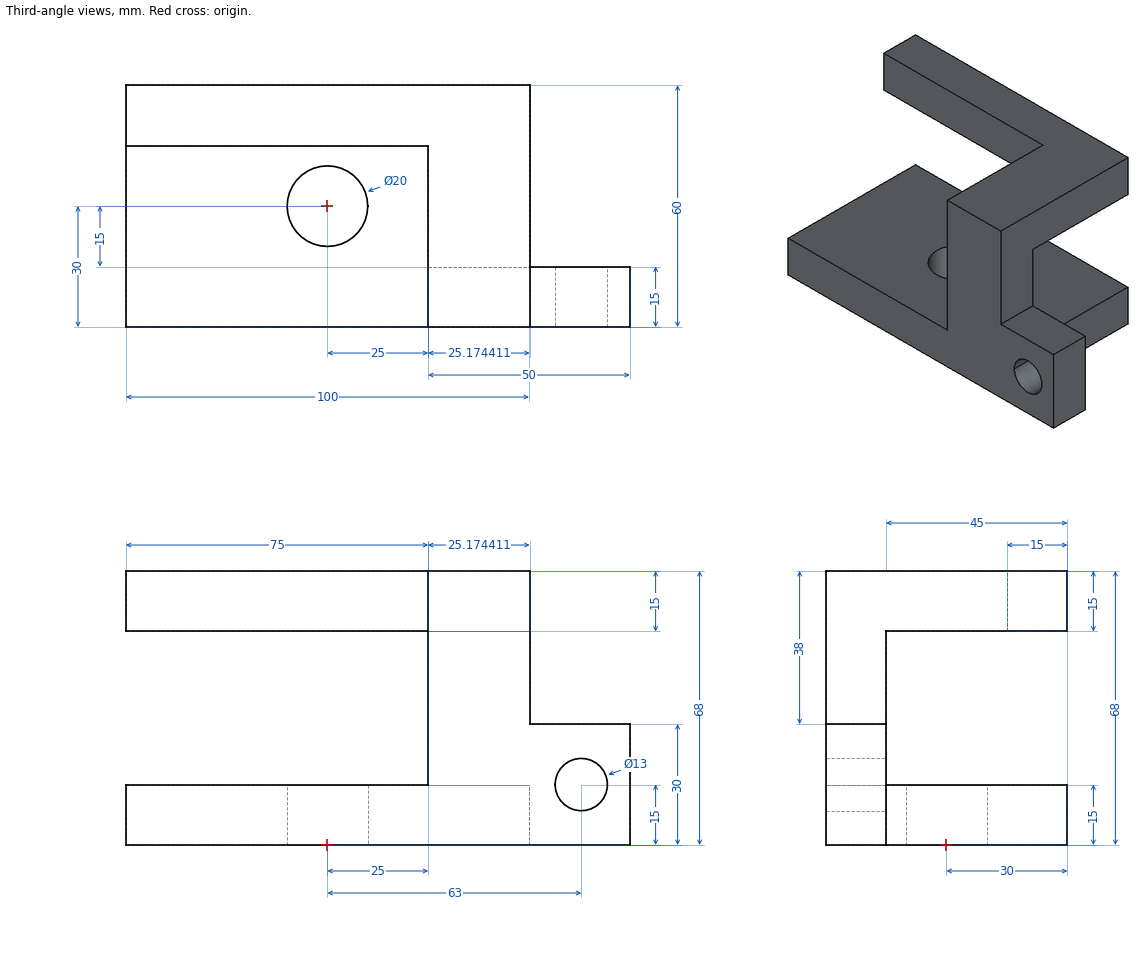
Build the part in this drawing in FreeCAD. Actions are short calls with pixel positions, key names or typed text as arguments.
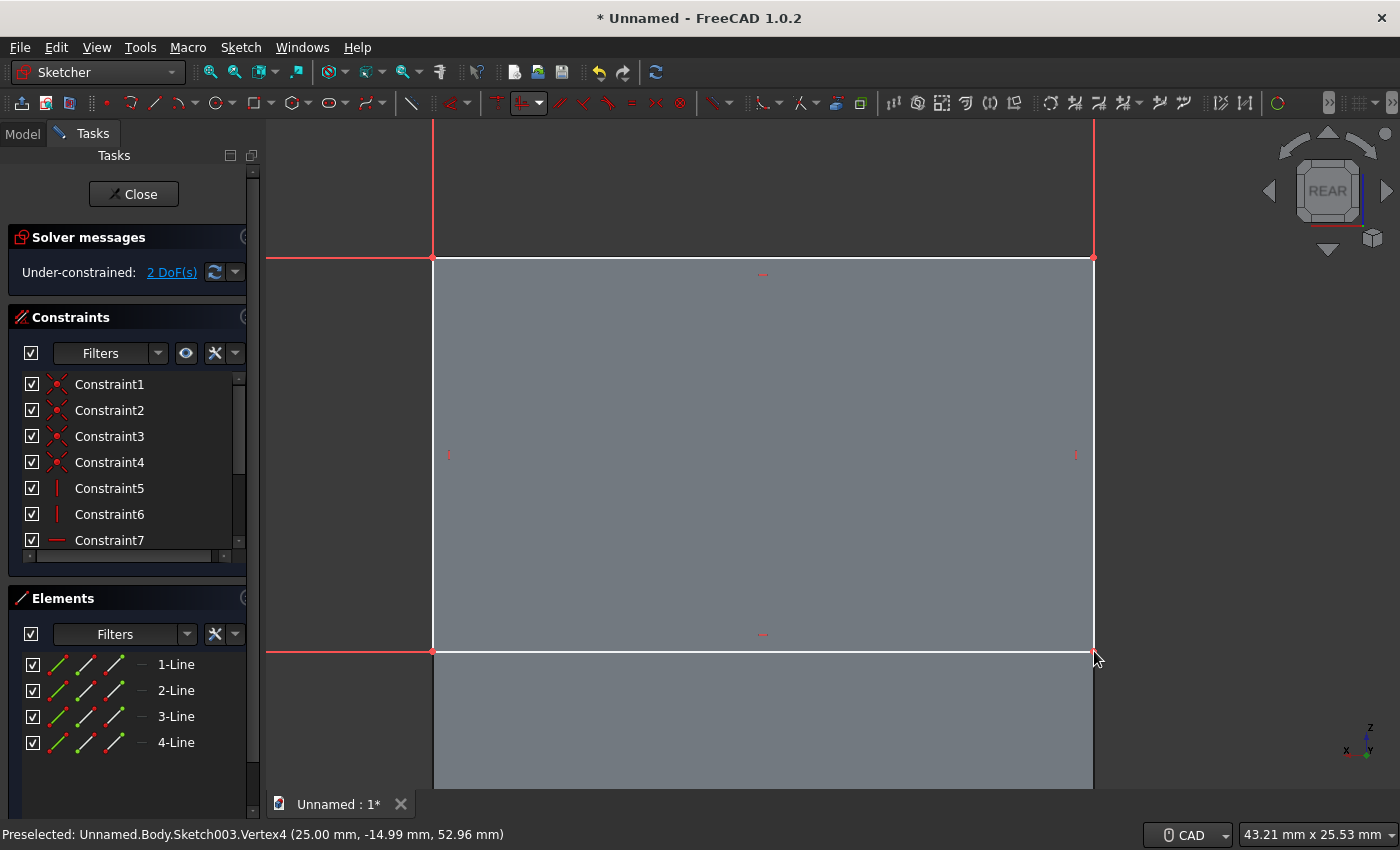
click(450, 104)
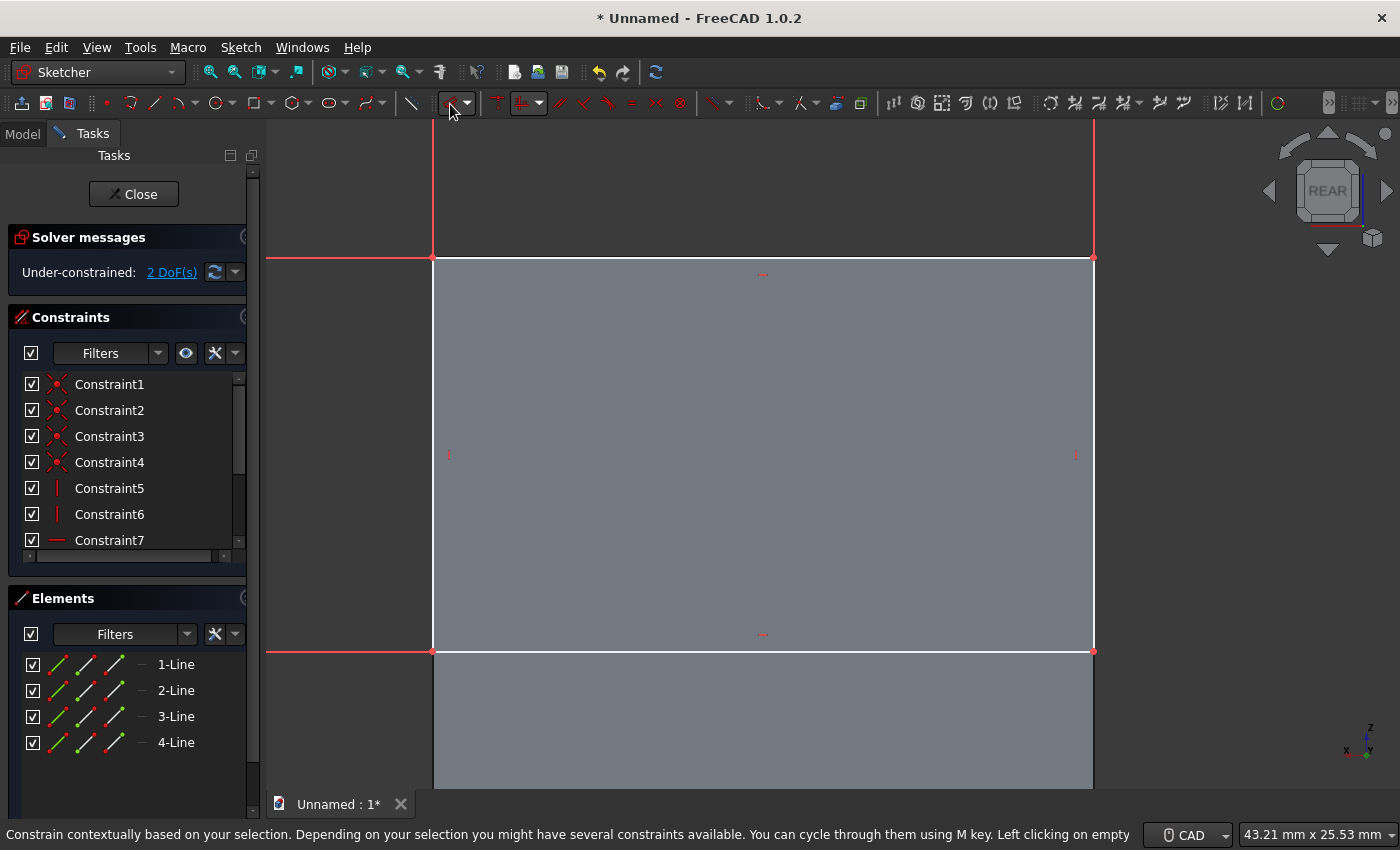
click(433, 258)
click(399, 510)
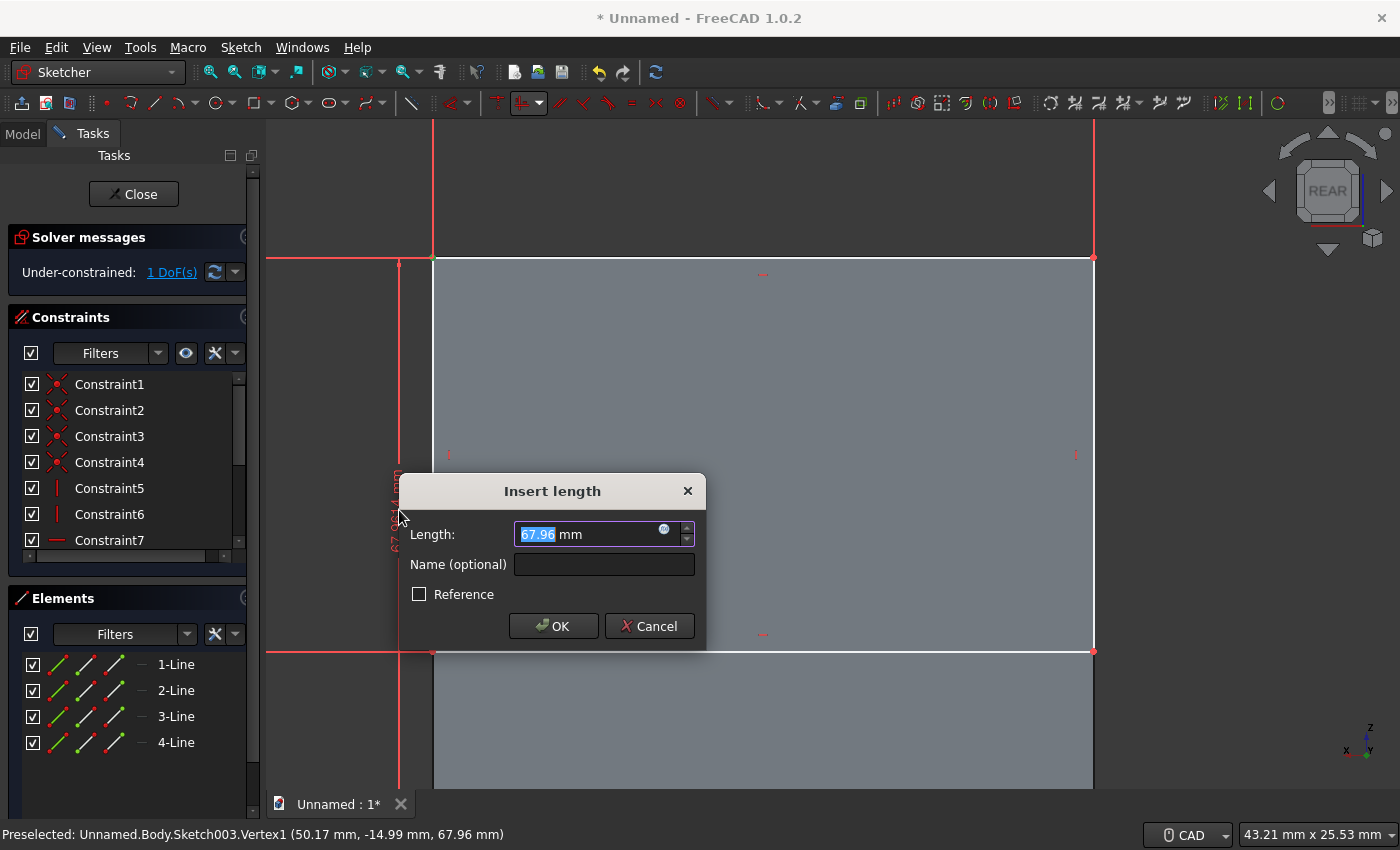
text(68)
key(Return)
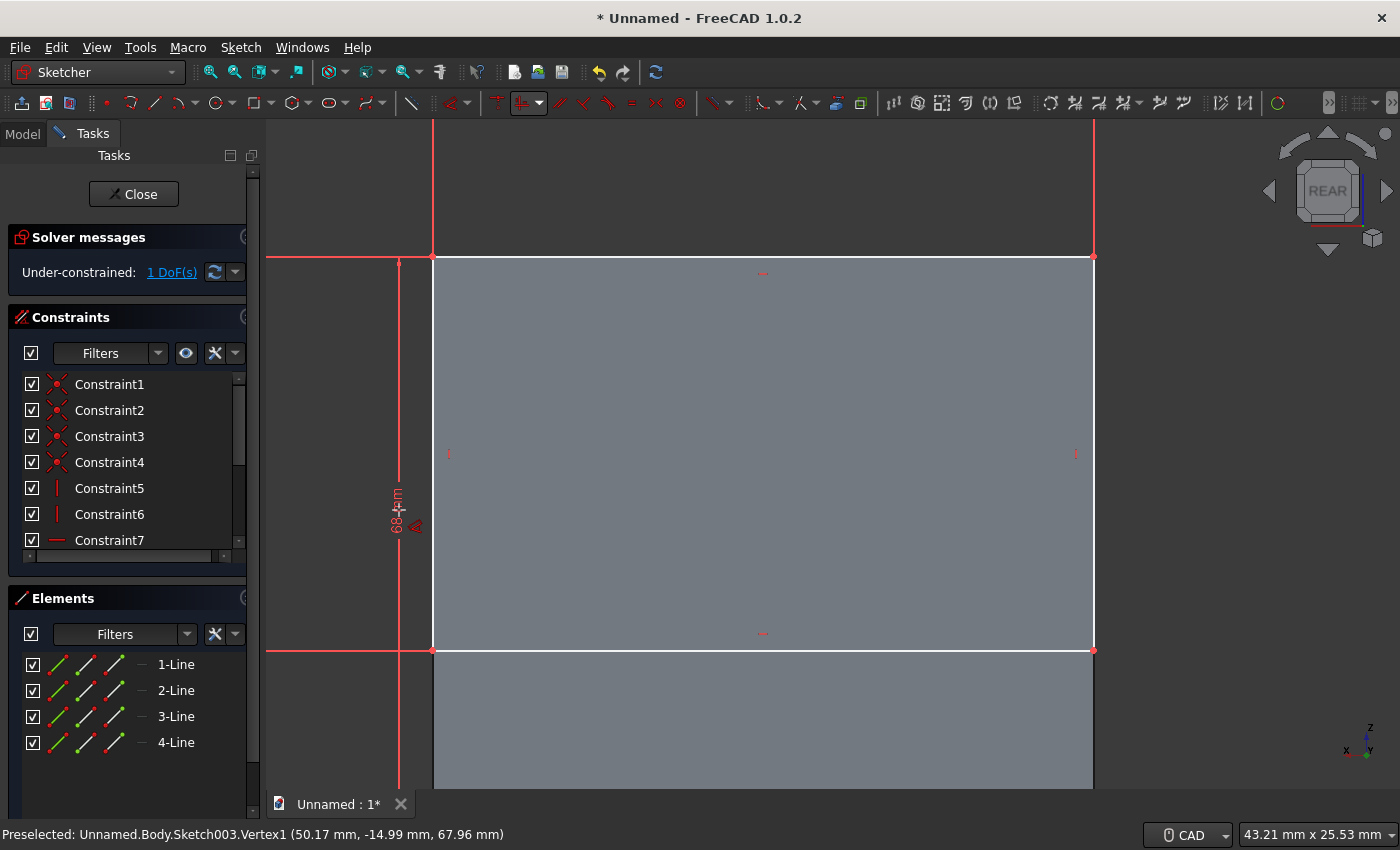
click(1094, 651)
click(1164, 617)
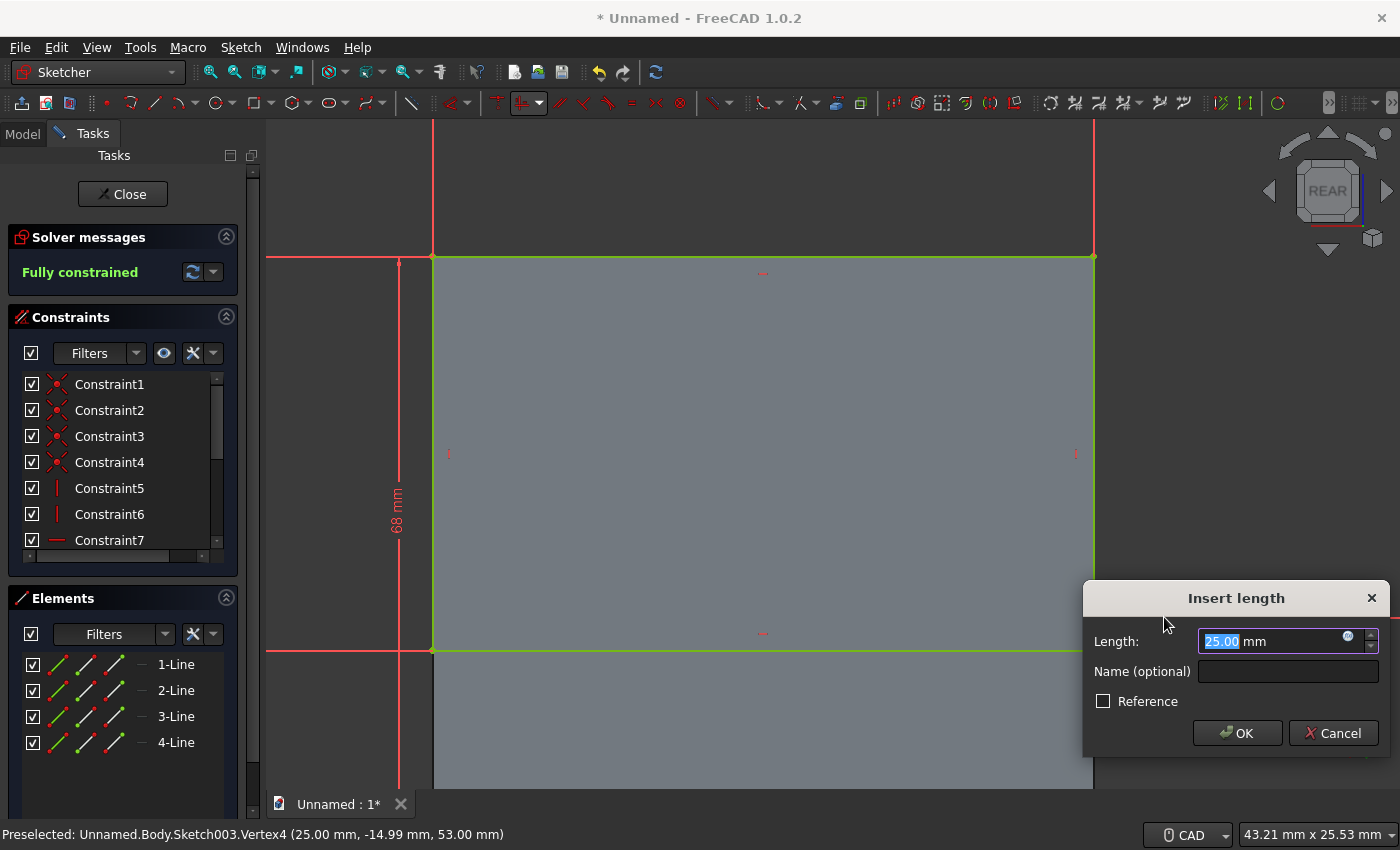
text(25)
key(Return)
key(Escape)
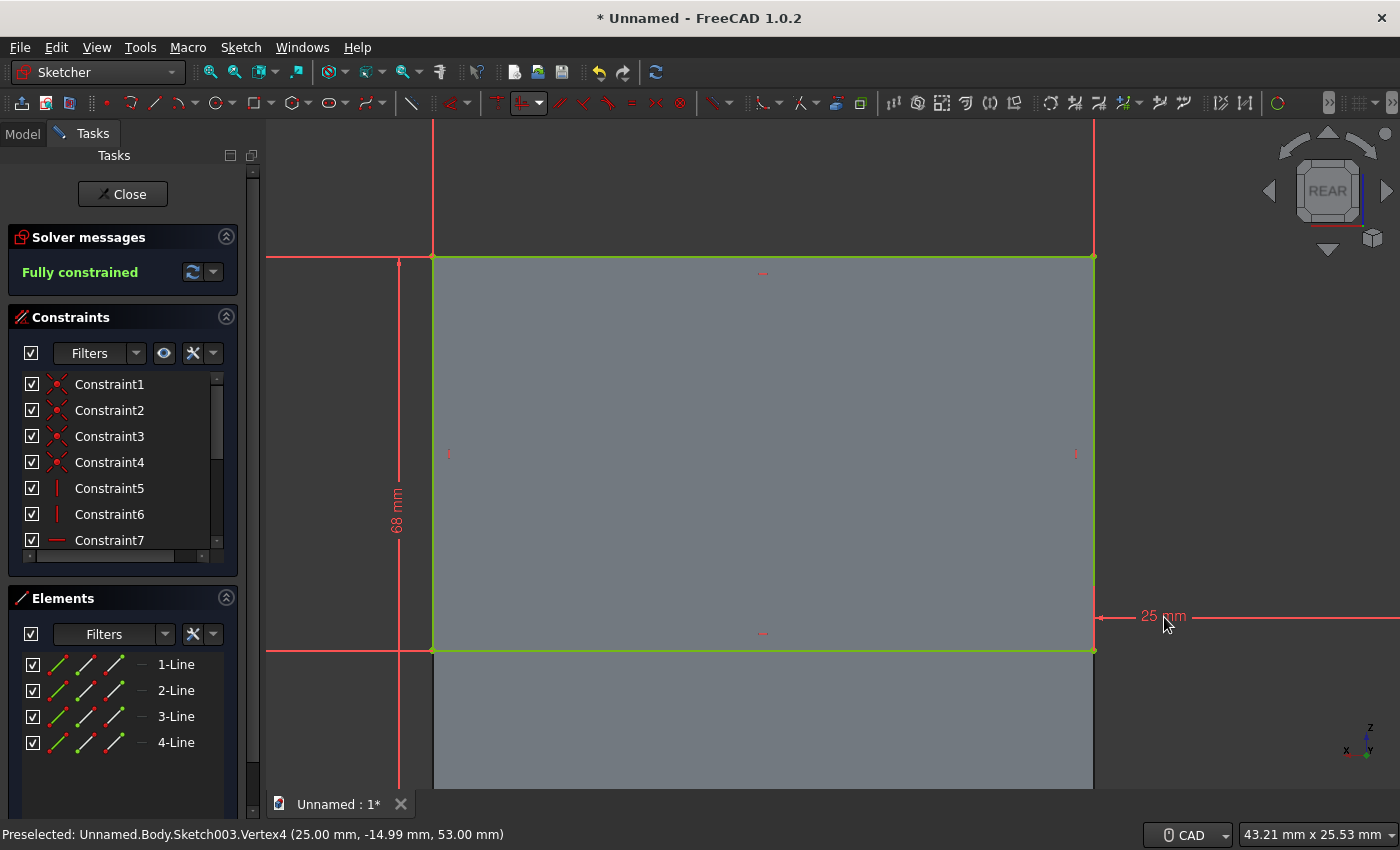
click(123, 194)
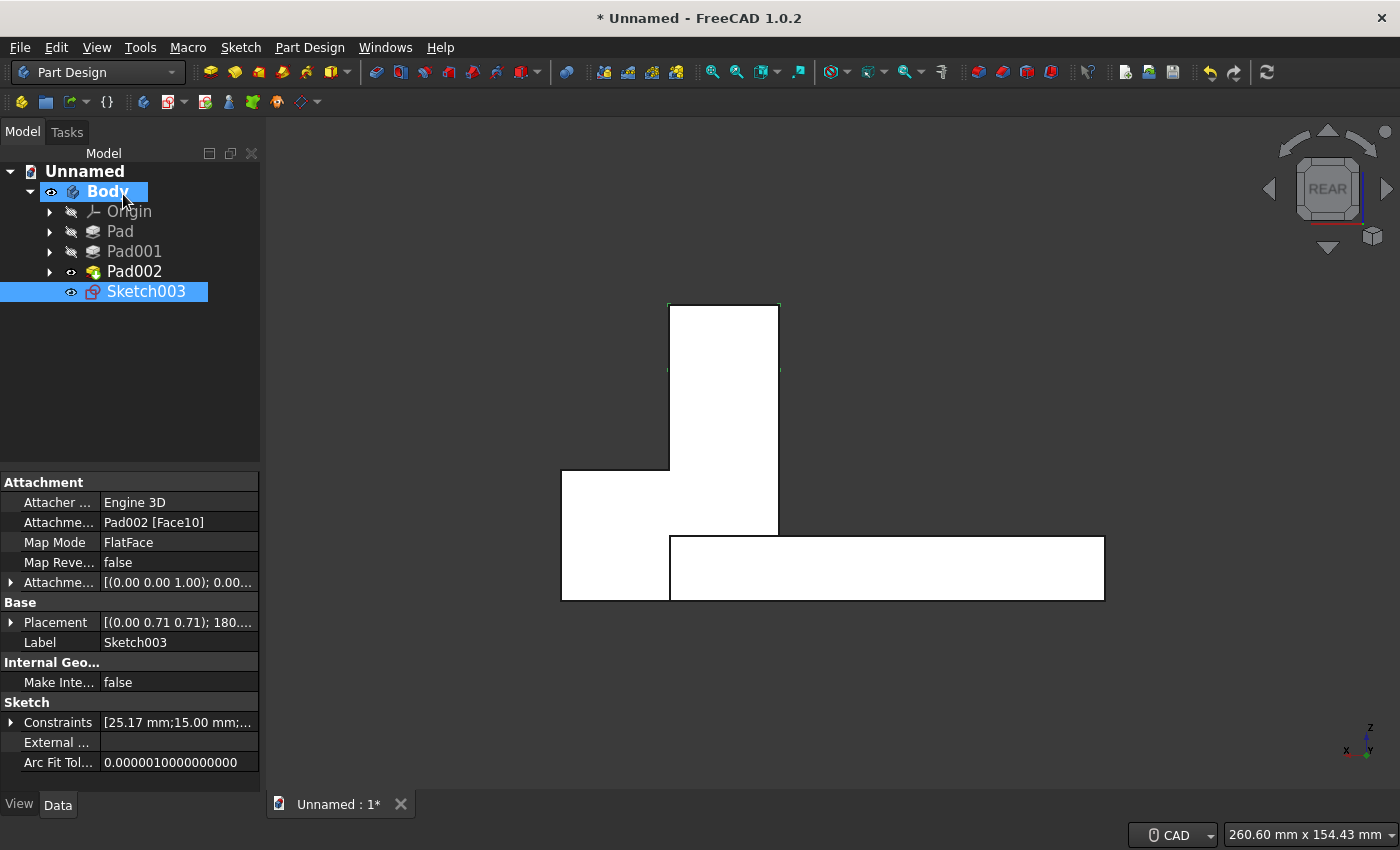
click(212, 72)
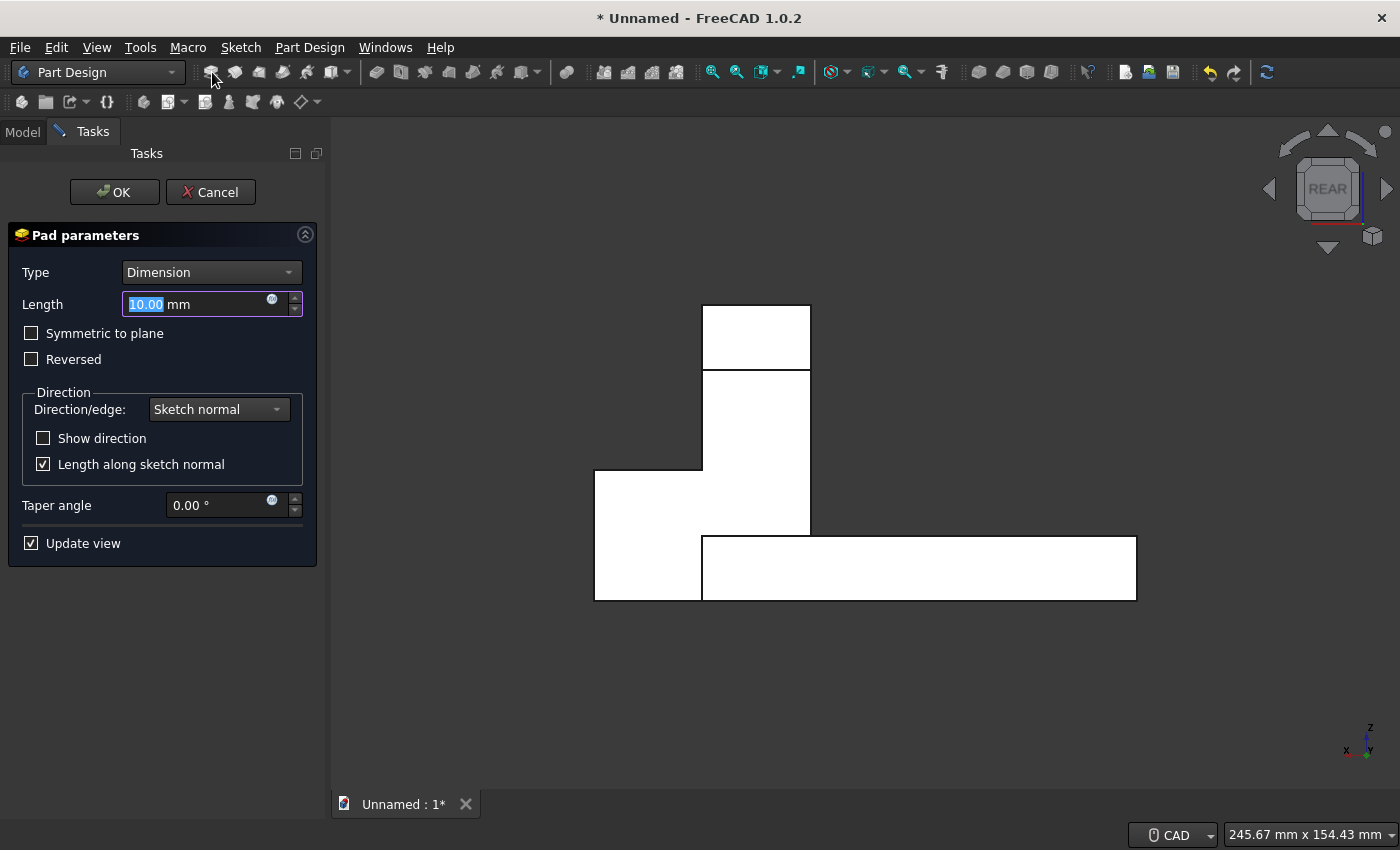
text(45)
key(Tab)